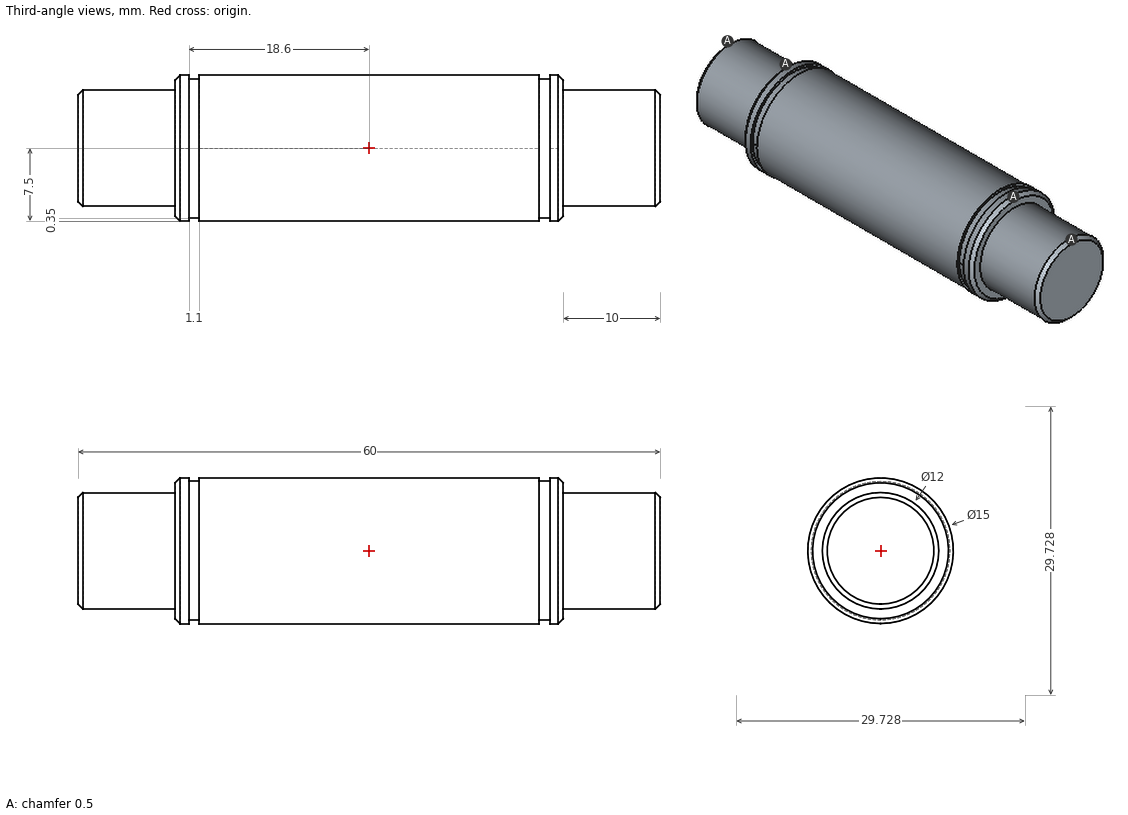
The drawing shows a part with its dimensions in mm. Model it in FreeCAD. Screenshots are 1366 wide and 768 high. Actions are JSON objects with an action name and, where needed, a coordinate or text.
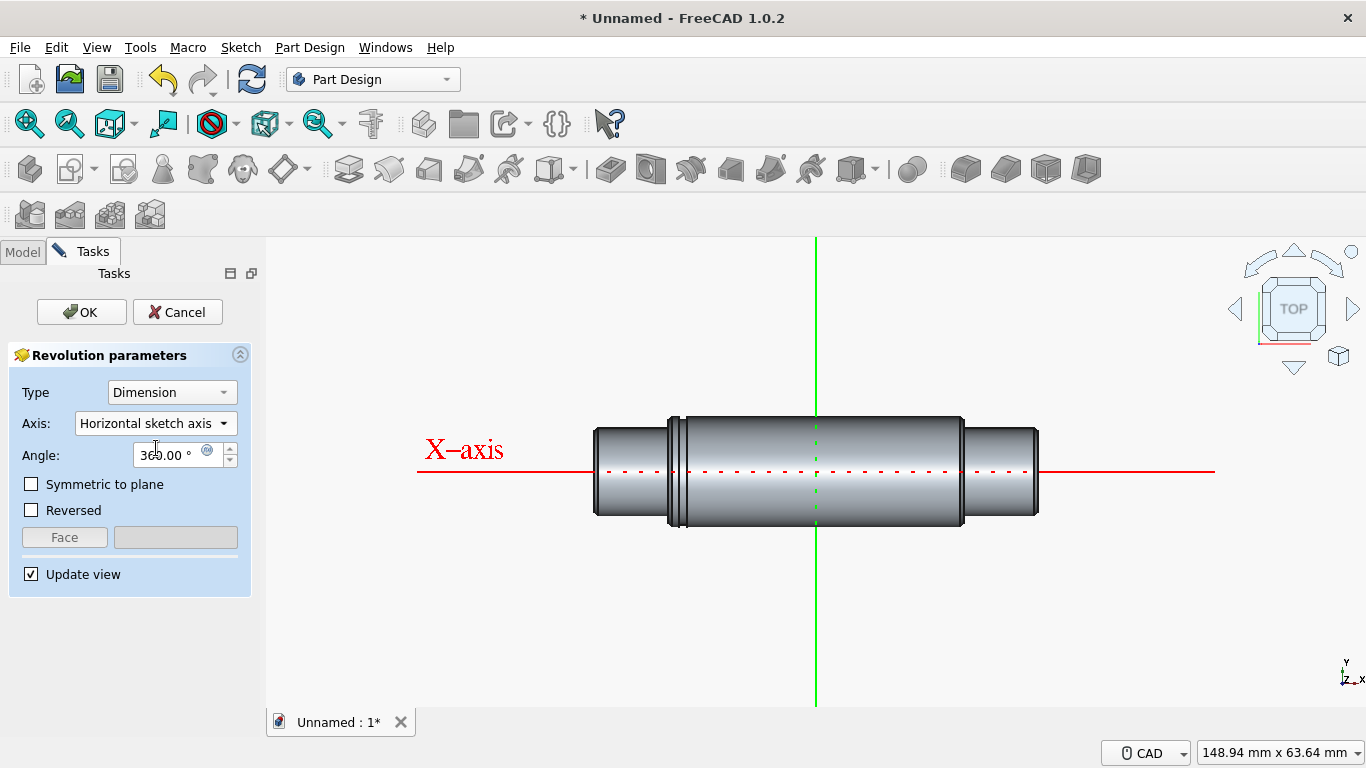
{"action": "left_click", "coordinate": [82, 312]}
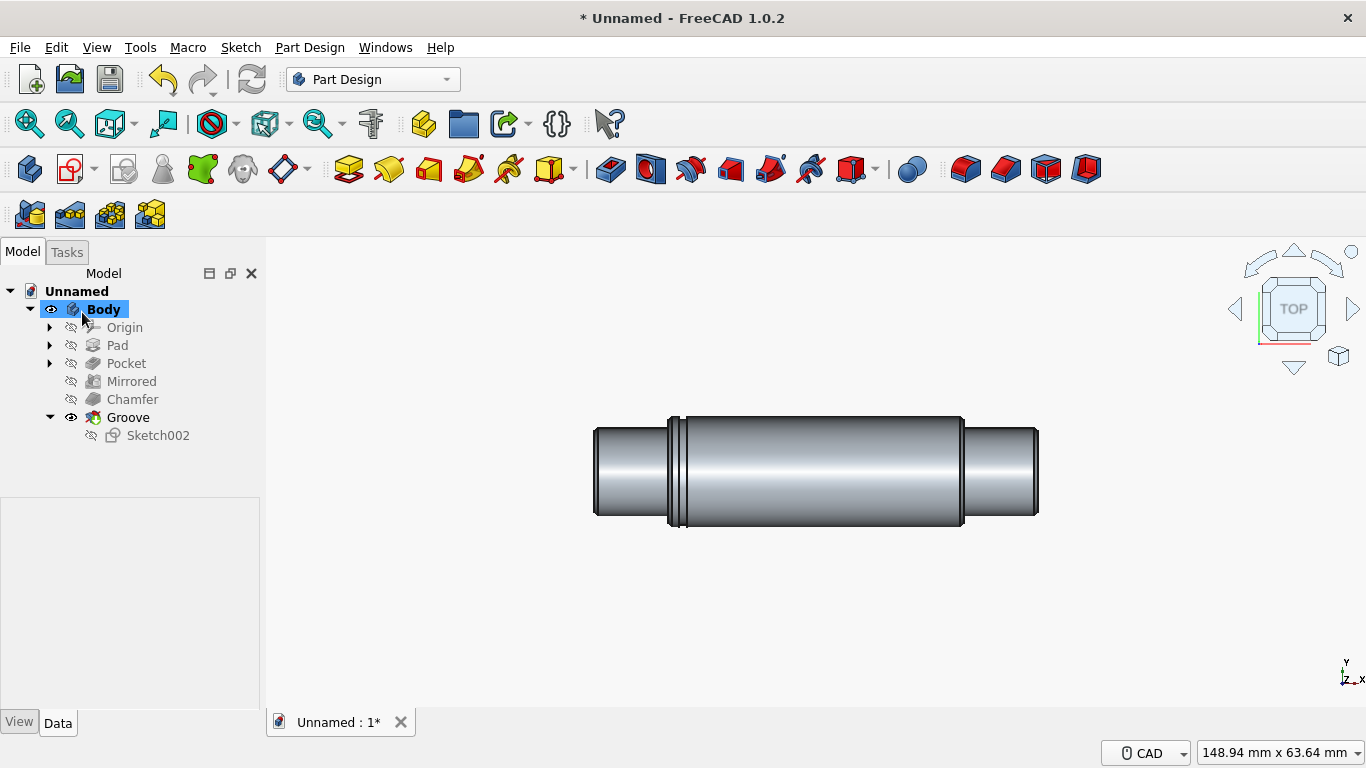
{"action": "key", "text": "v f"}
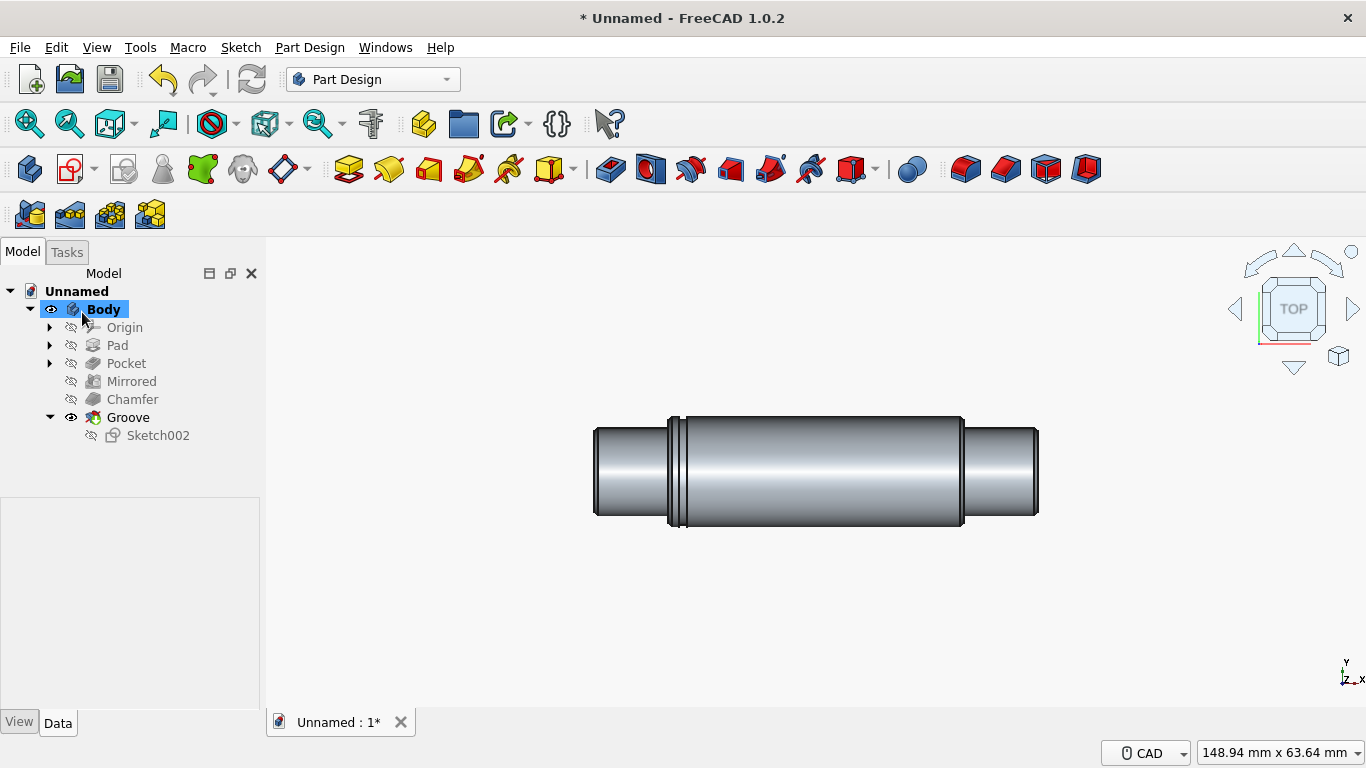
{"action": "left_click", "coordinate": [116, 417]}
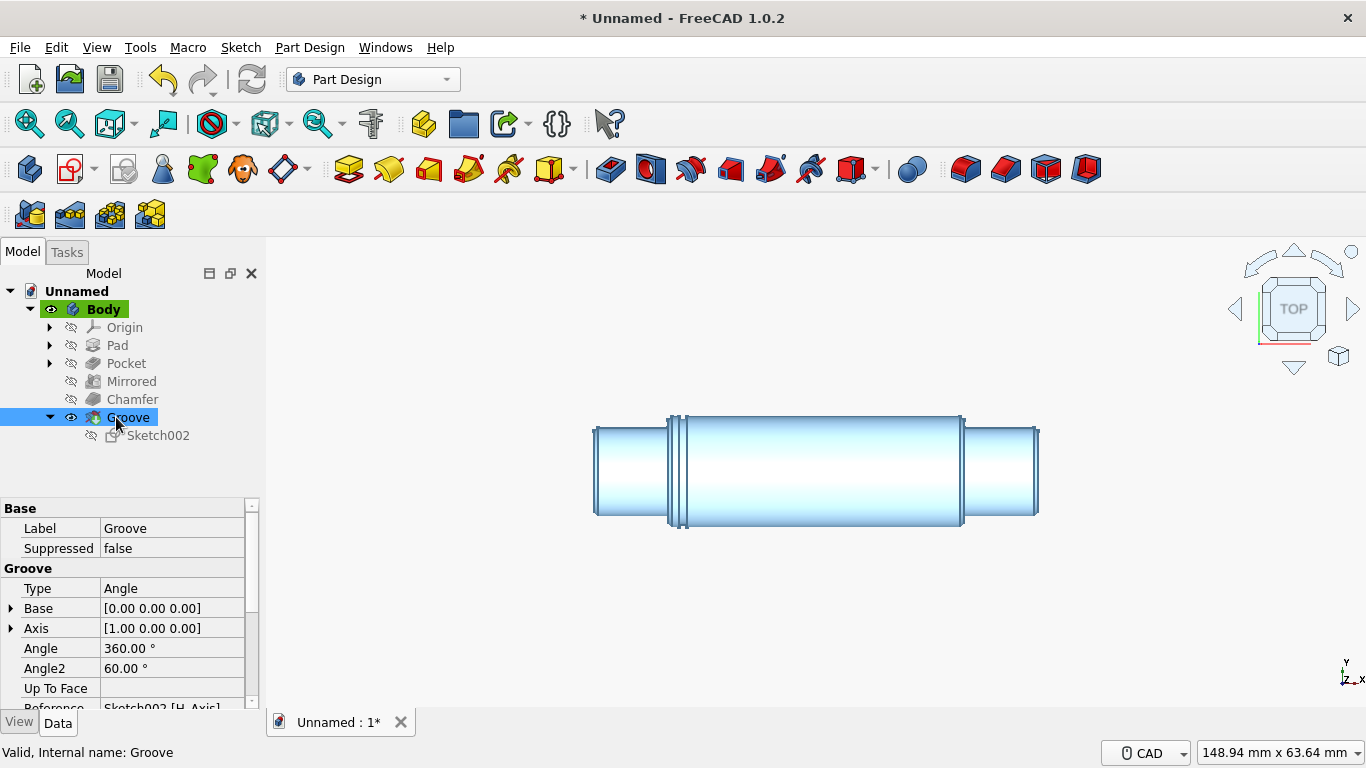
{"action": "left_click", "coordinate": [30, 214]}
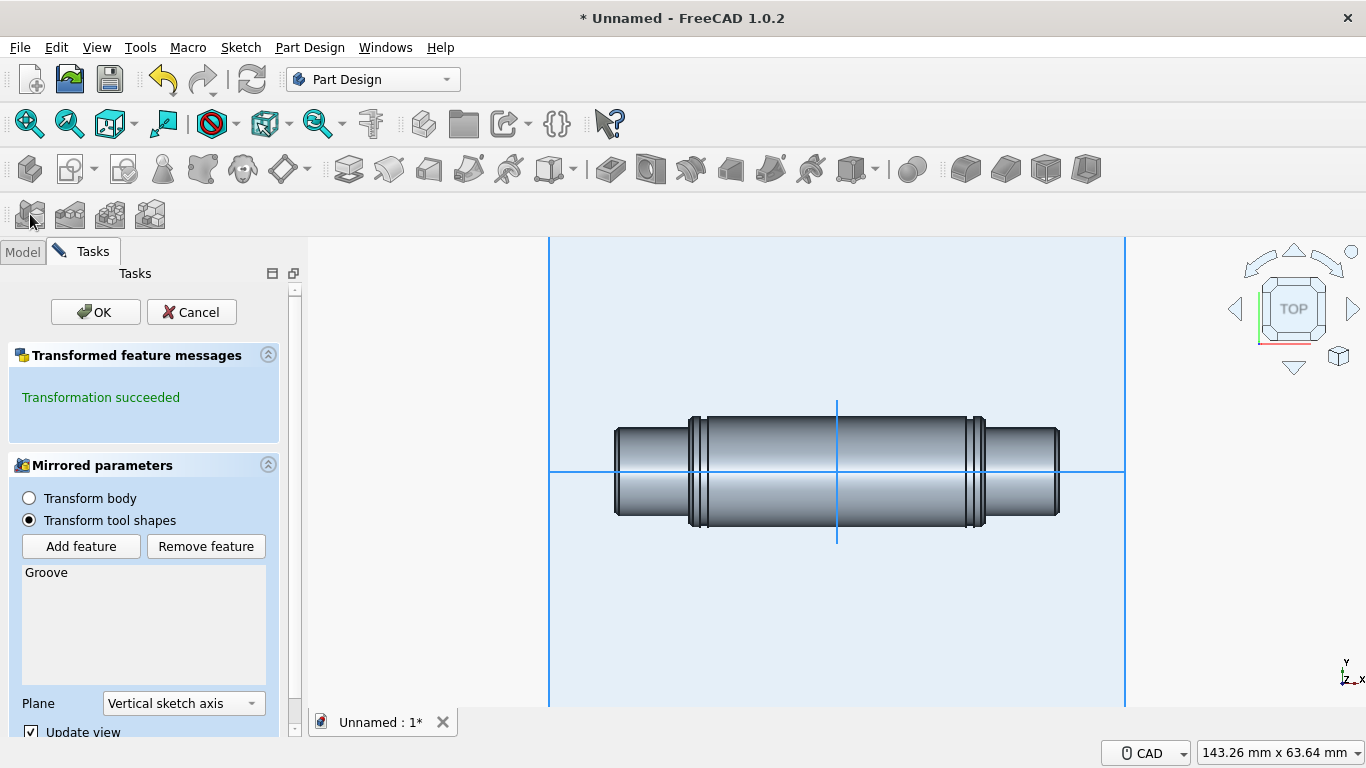
{"action": "left_click", "coordinate": [184, 704]}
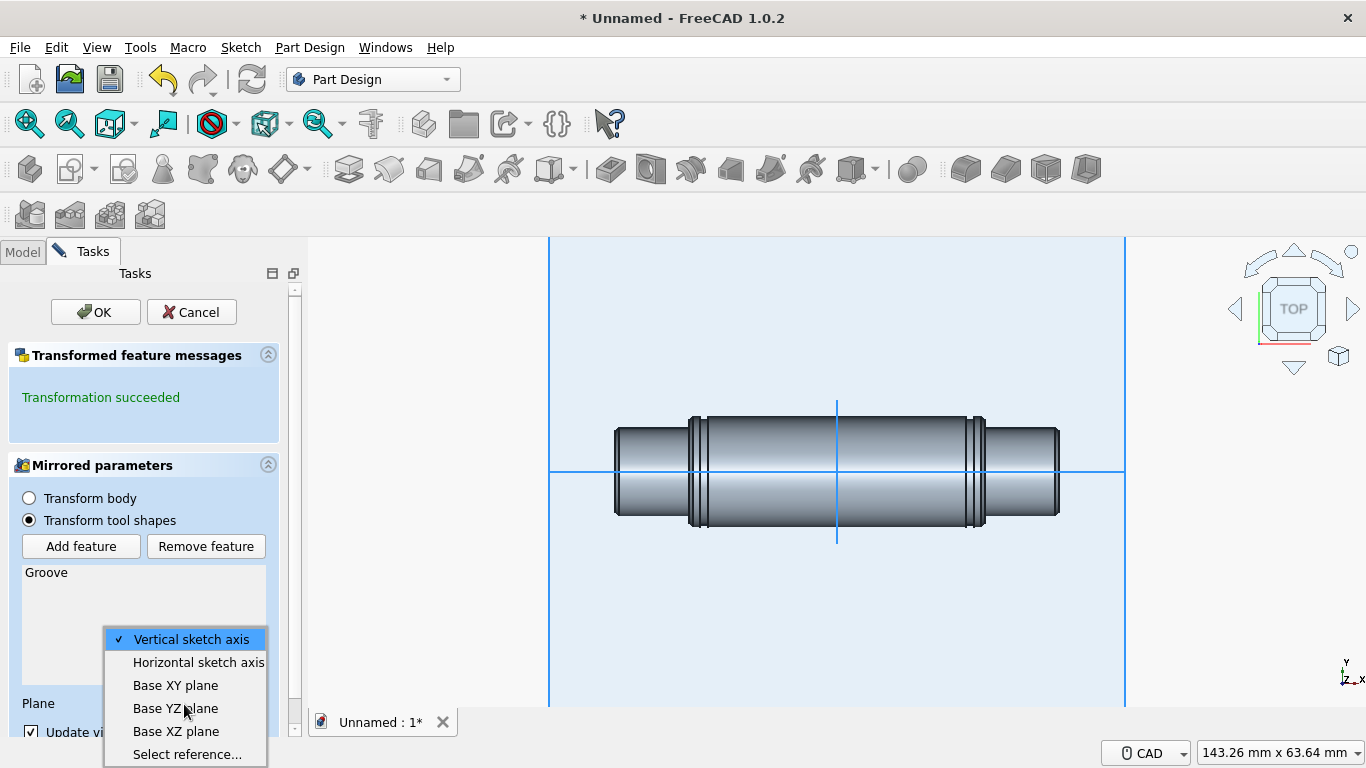
{"action": "left_click", "coordinate": [184, 708]}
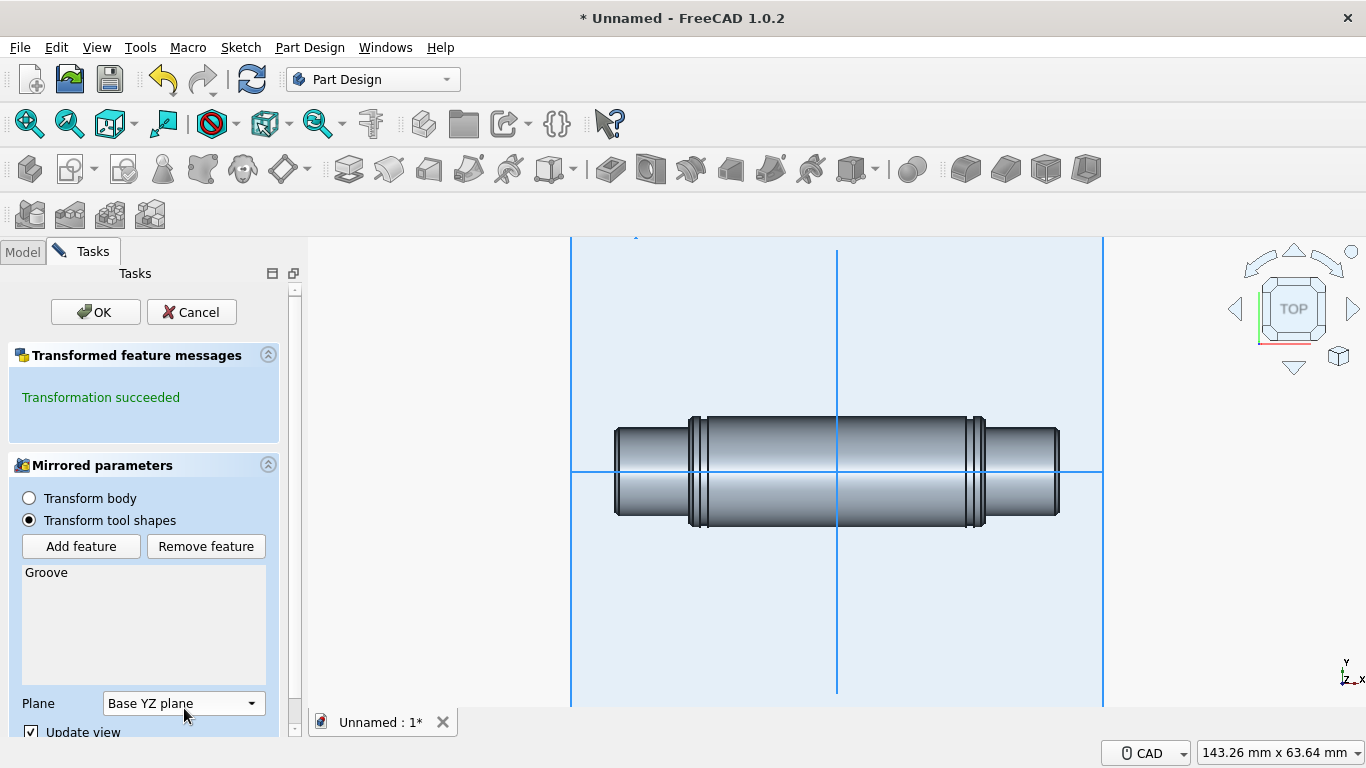
{"action": "left_click", "coordinate": [96, 312]}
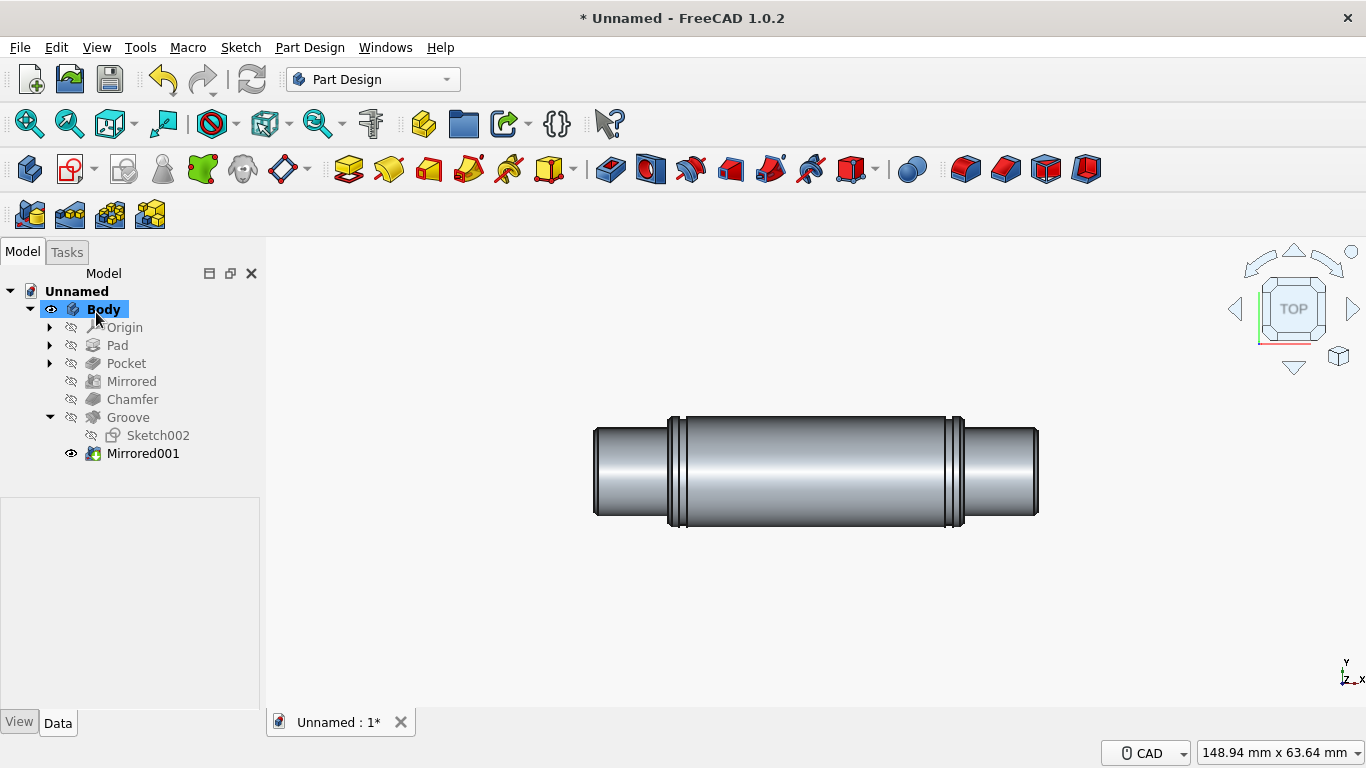
{"action": "key", "text": "0"}